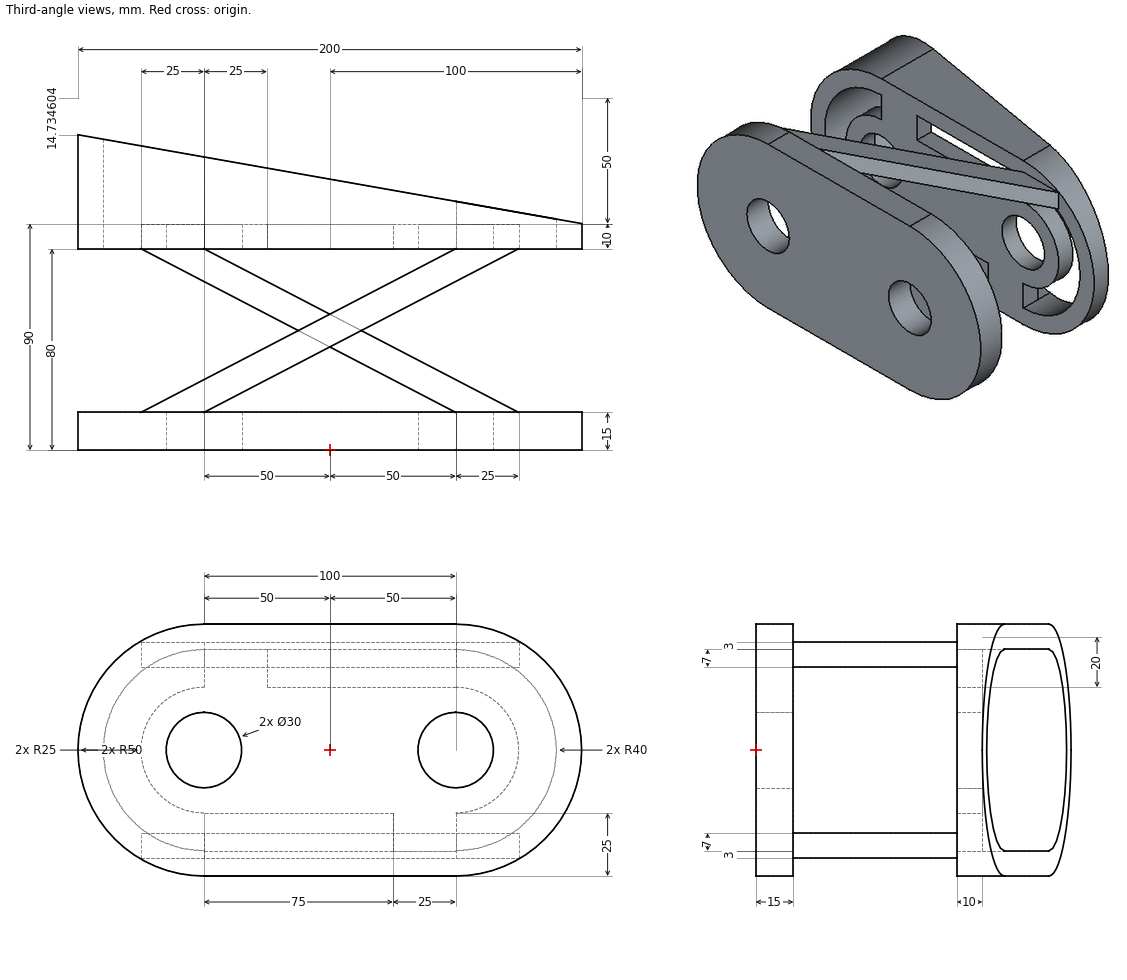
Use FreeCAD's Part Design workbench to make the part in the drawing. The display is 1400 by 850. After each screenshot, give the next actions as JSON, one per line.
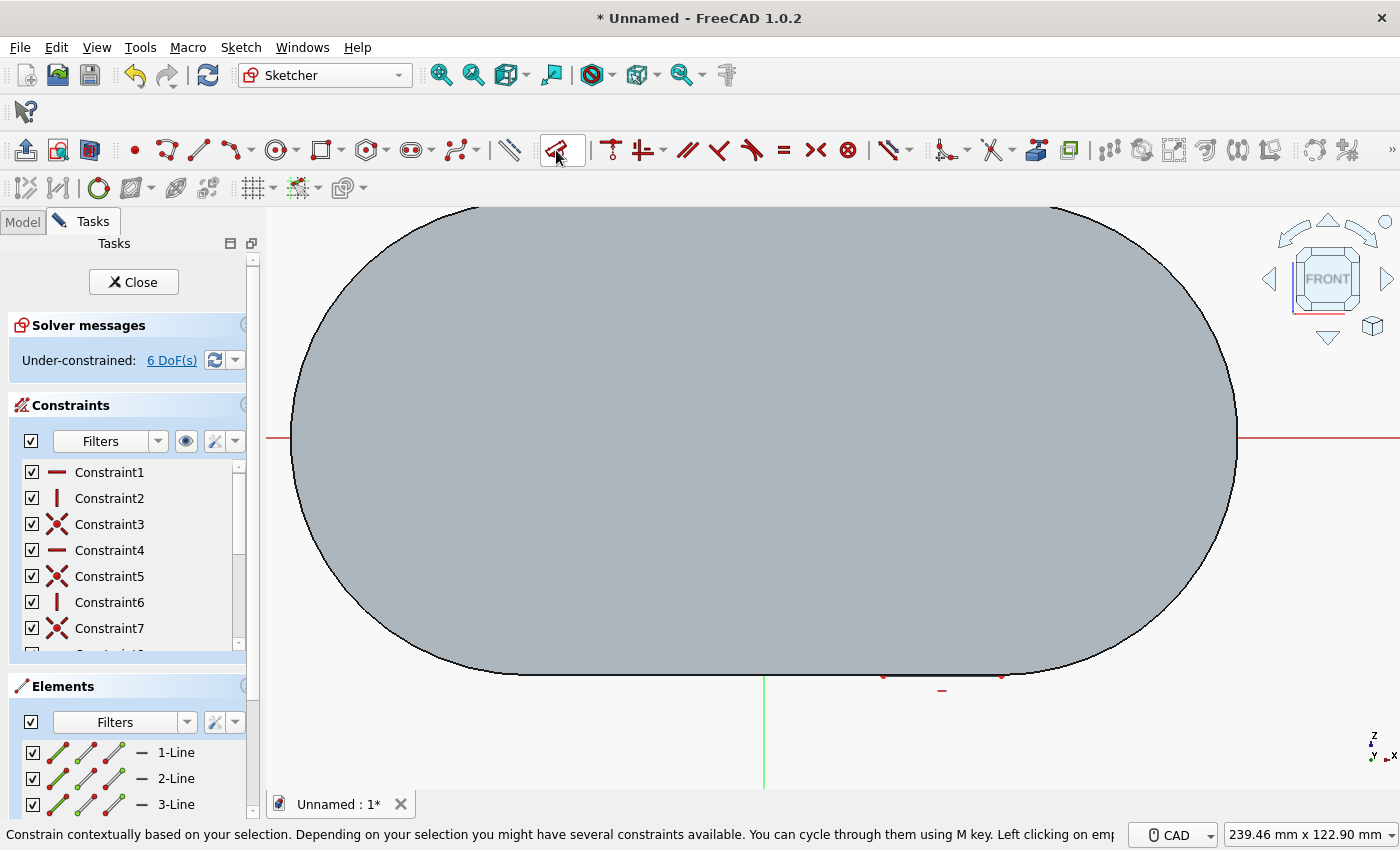
{"action": "left_click", "coordinate": [1098, 509]}
{"action": "left_click", "coordinate": [1124, 528]}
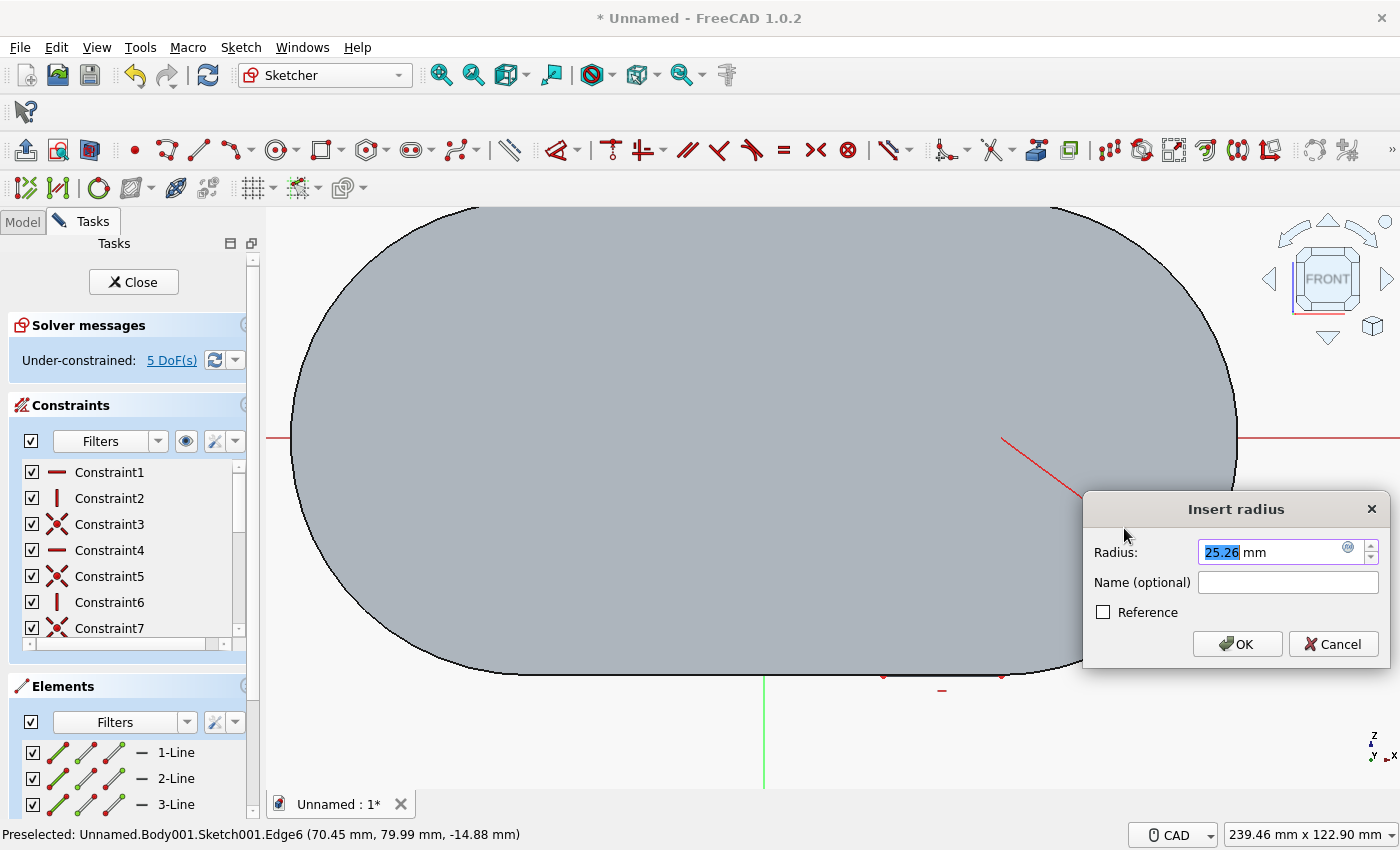
{"action": "type", "text": "25"}
{"action": "key", "text": "Return"}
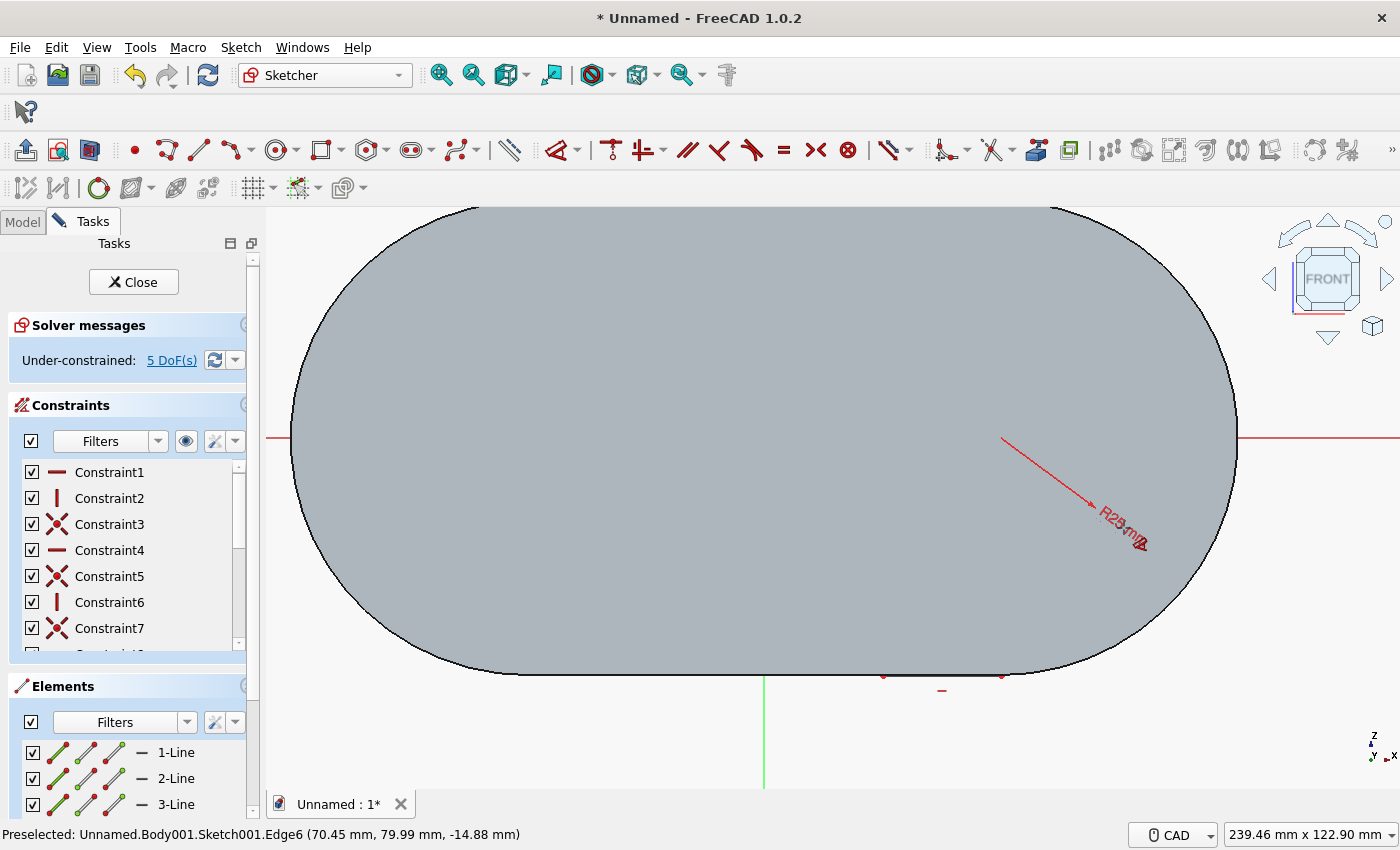
{"action": "left_click", "coordinate": [1001, 592]}
{"action": "left_click", "coordinate": [1035, 616]}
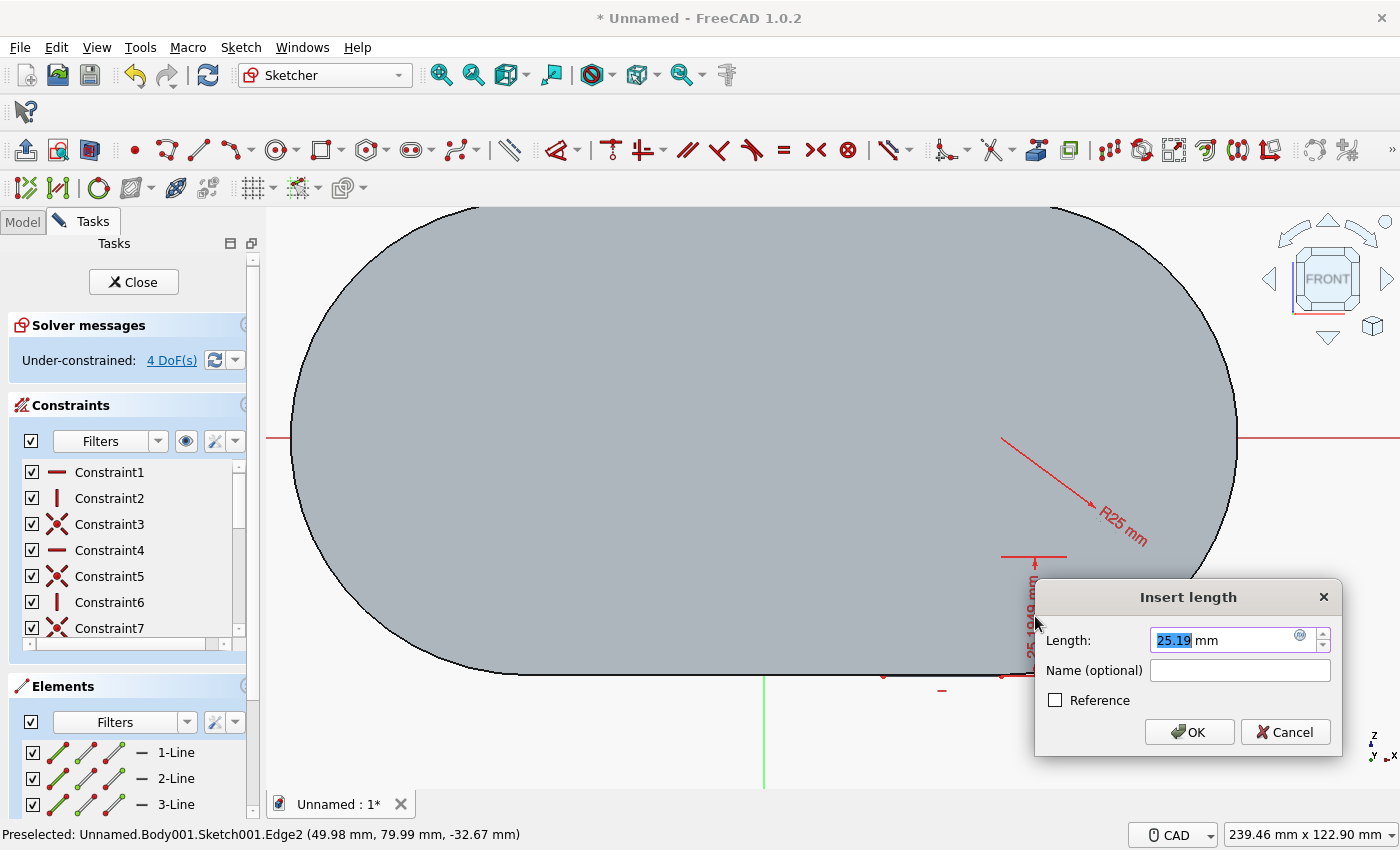
{"action": "type", "text": "25"}
{"action": "key", "text": "Return"}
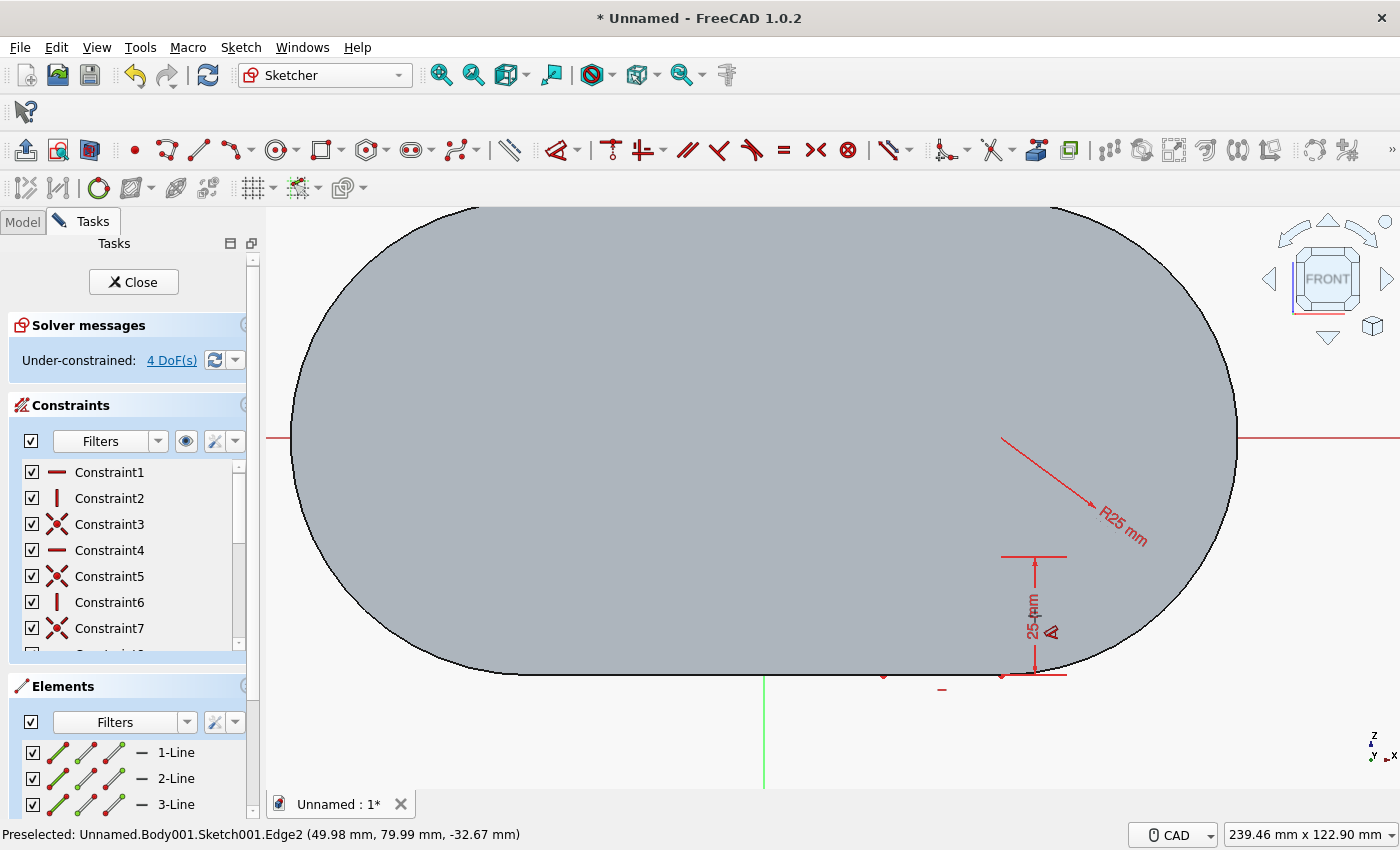
{"action": "left_click", "coordinate": [966, 675]}
{"action": "left_click", "coordinate": [942, 709]}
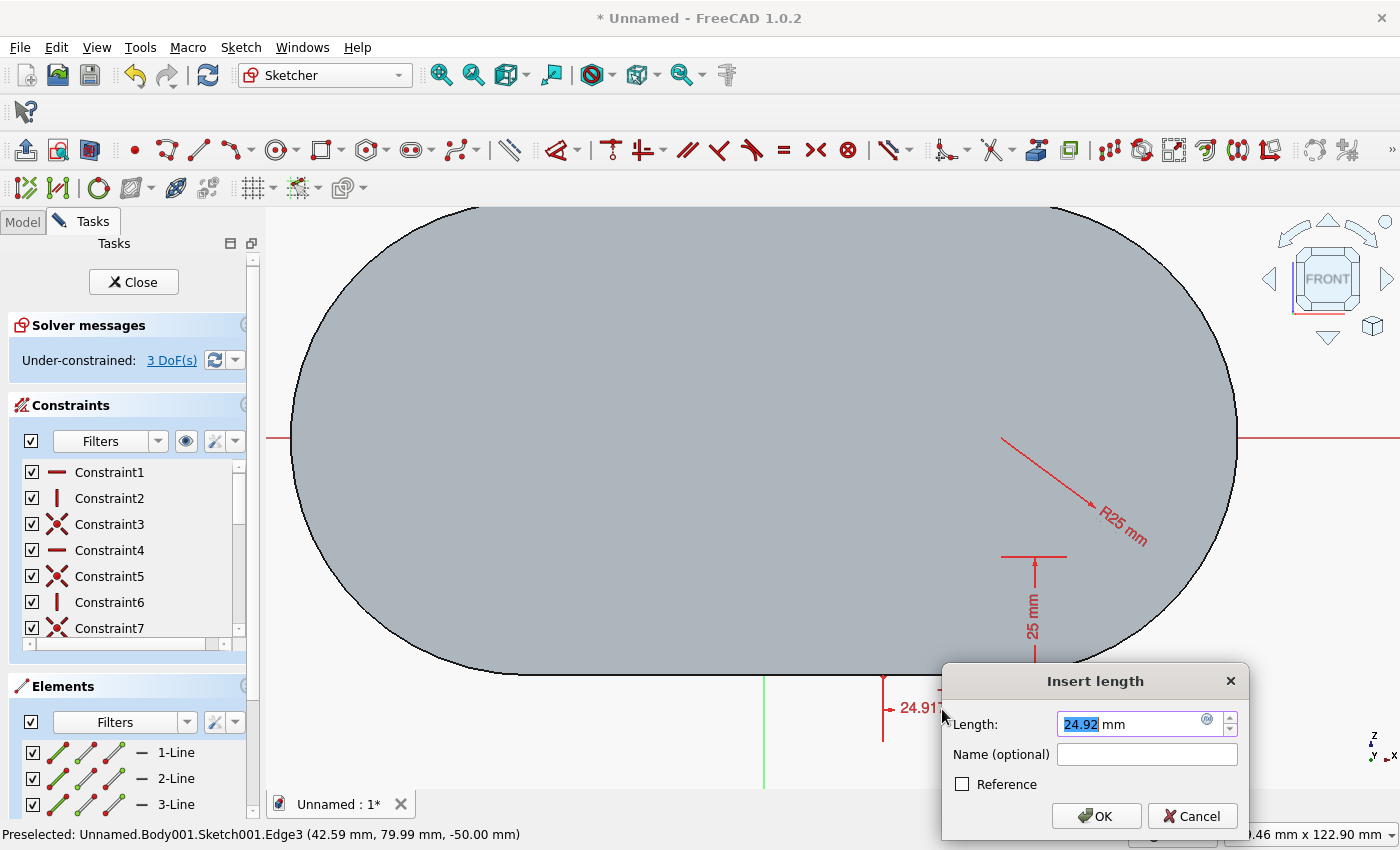
{"action": "type", "text": "25"}
{"action": "key", "text": "Return"}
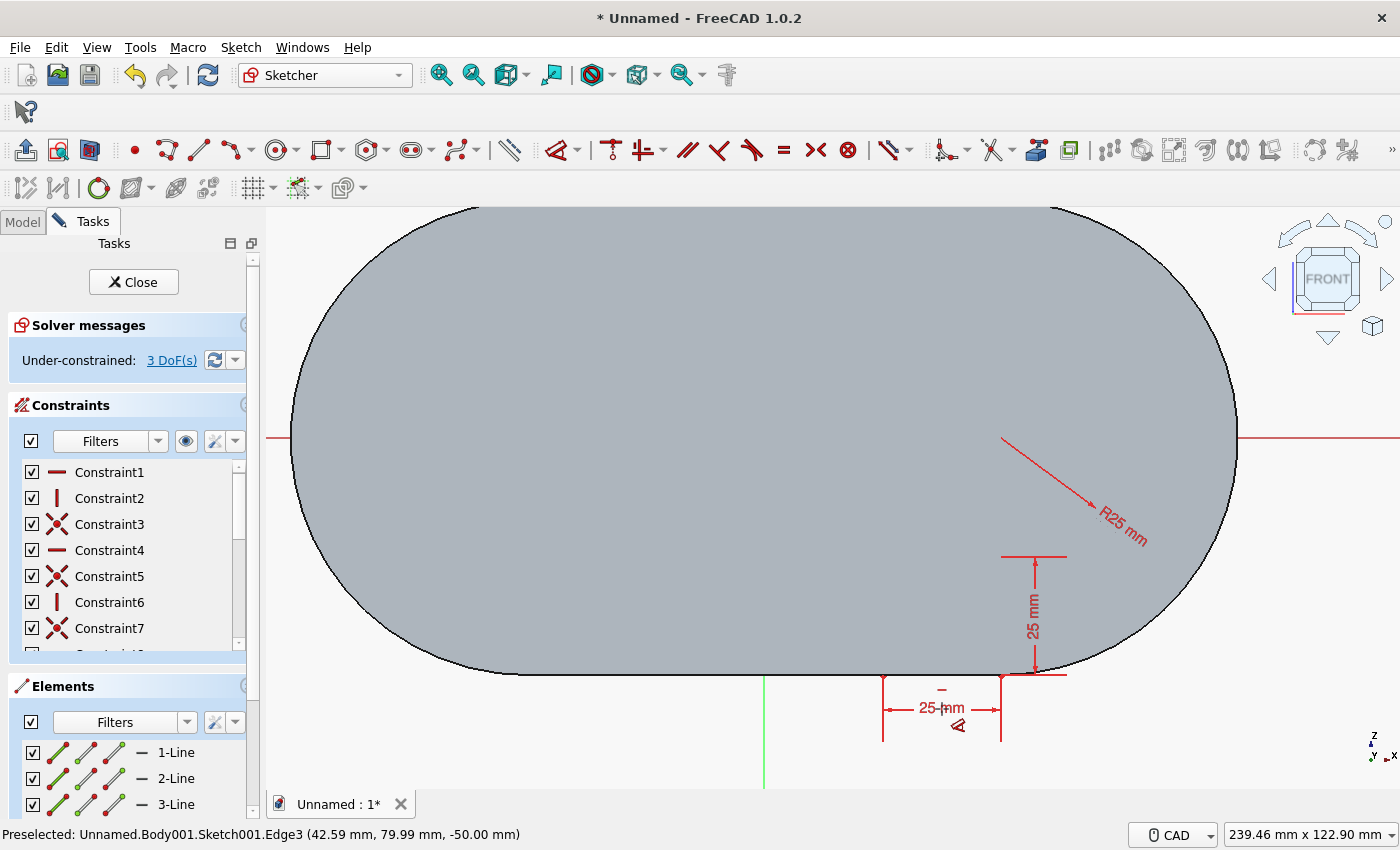
{"action": "left_click", "coordinate": [776, 557]}
{"action": "left_click", "coordinate": [705, 591]}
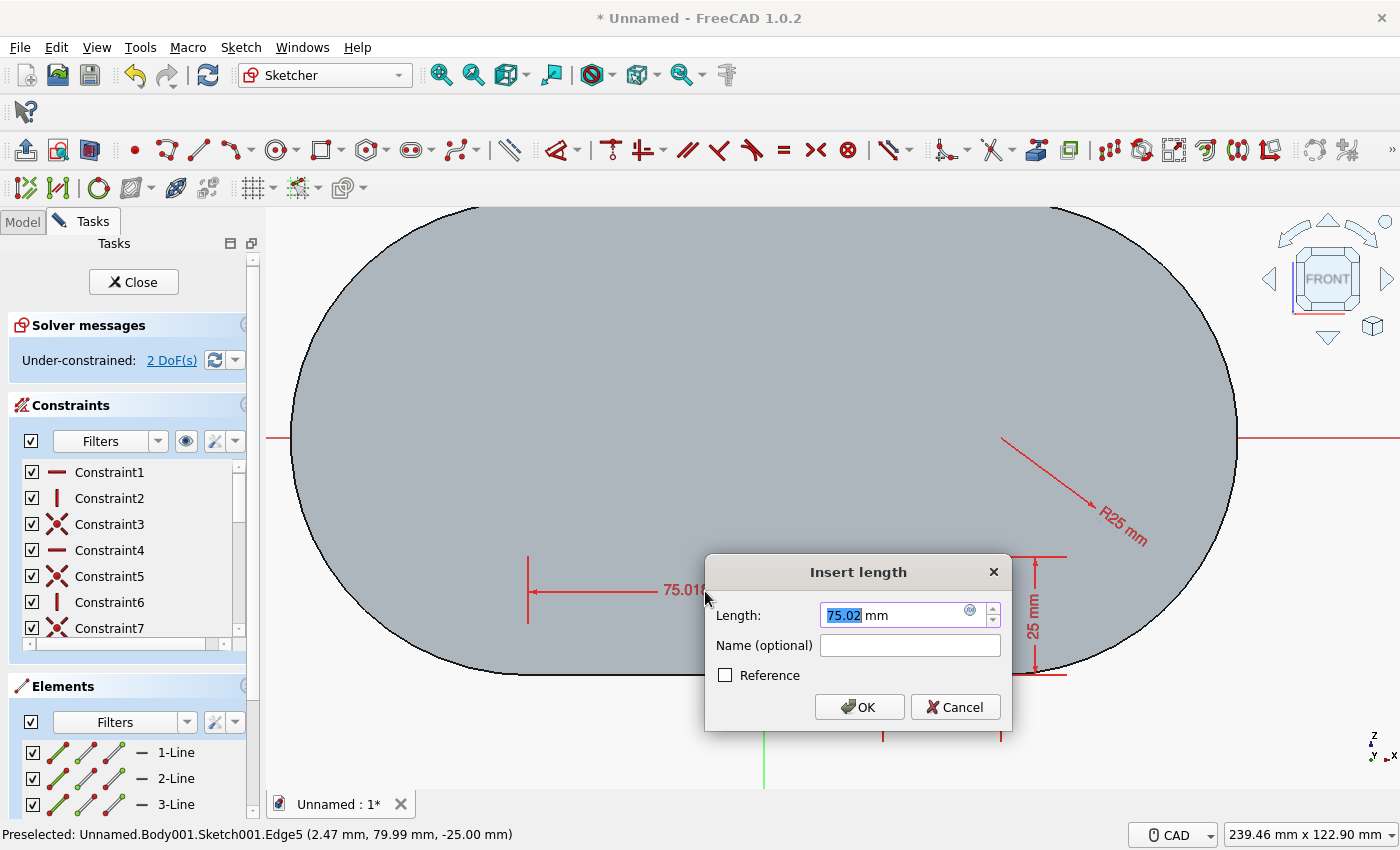
{"action": "type", "text": "75"}
{"action": "key", "text": "Return"}